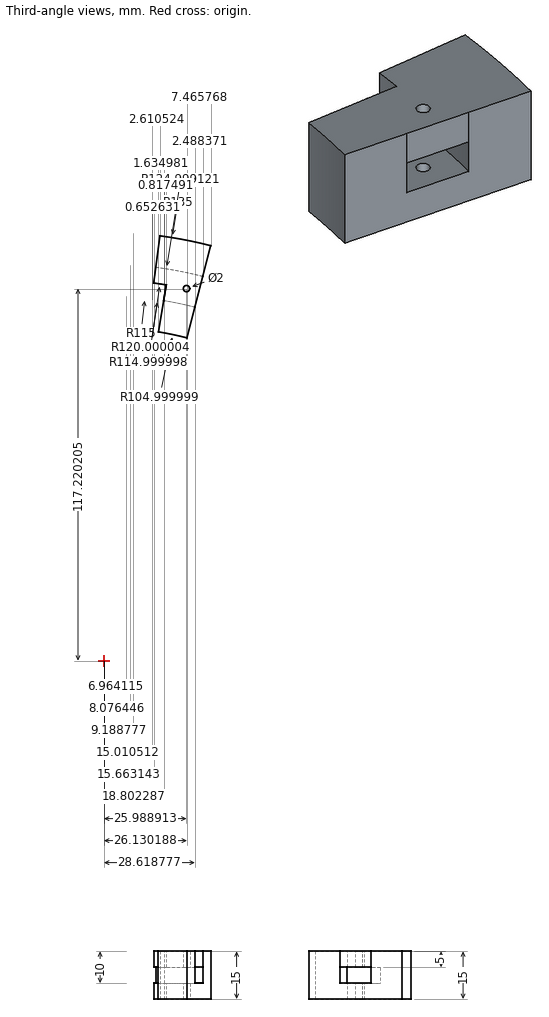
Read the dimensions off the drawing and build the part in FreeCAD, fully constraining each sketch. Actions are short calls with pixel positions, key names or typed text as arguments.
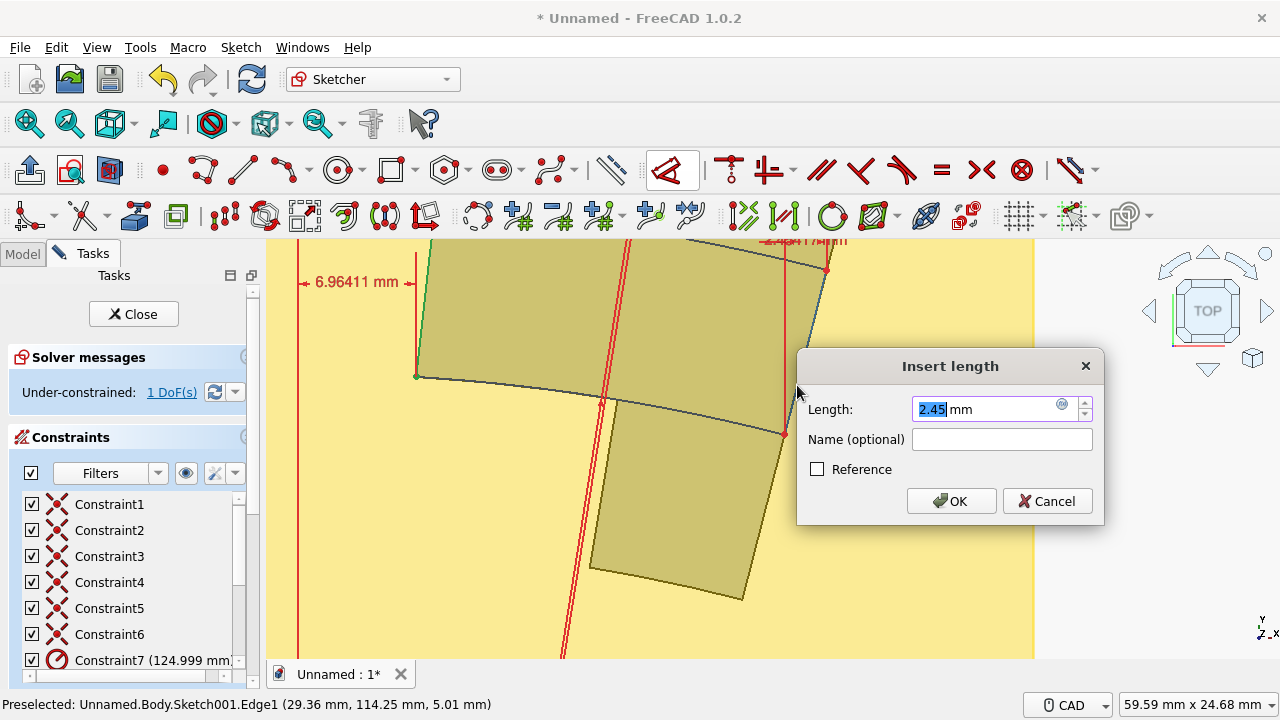
text(2.488371)
key(Return)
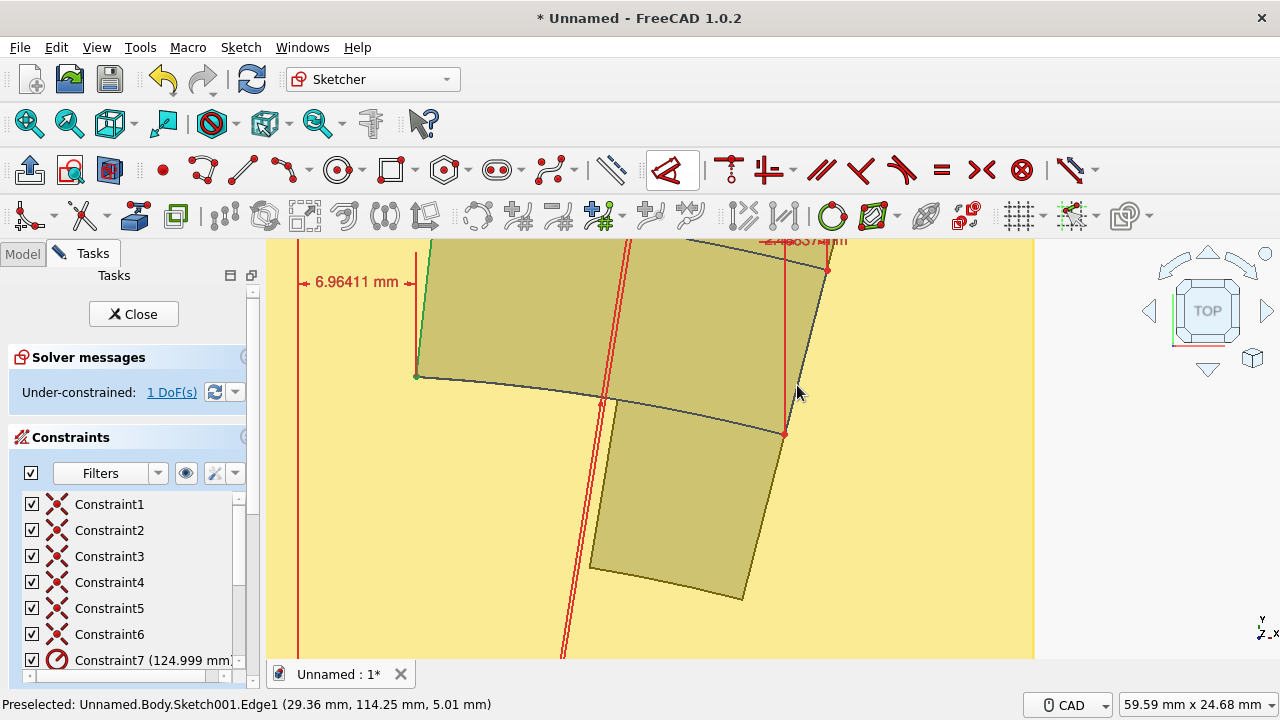
click(785, 435)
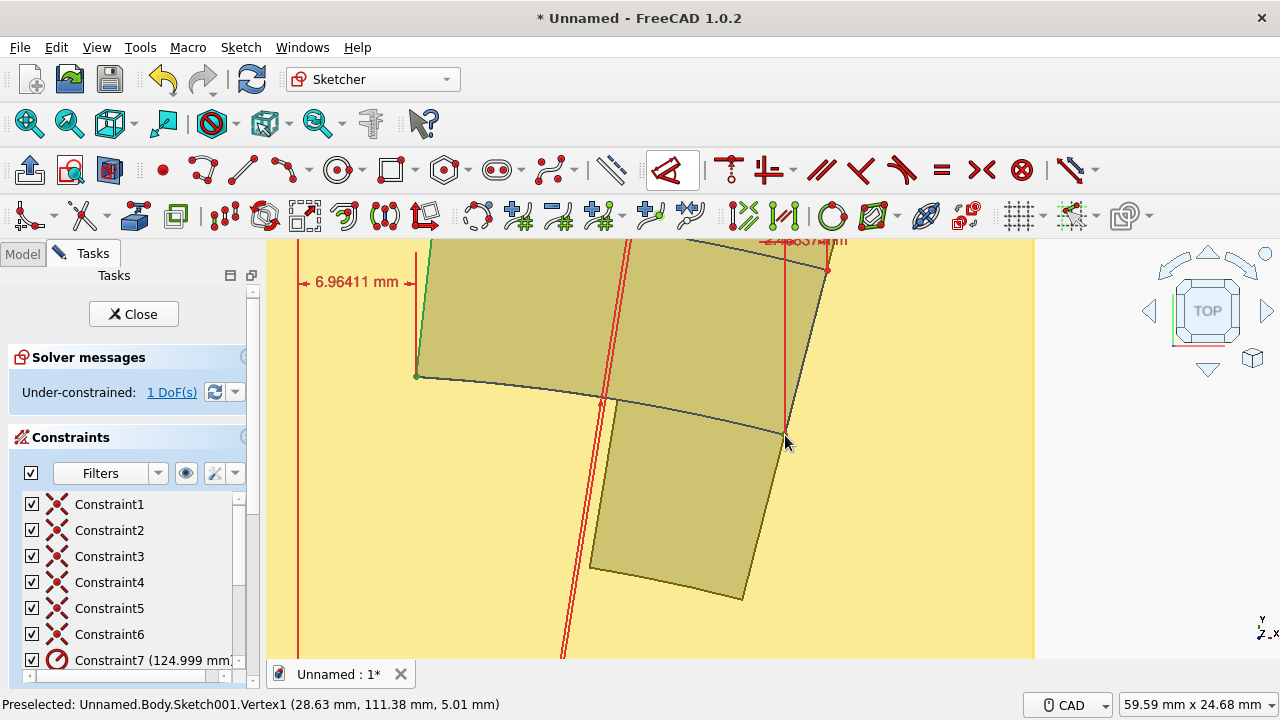
click(694, 170)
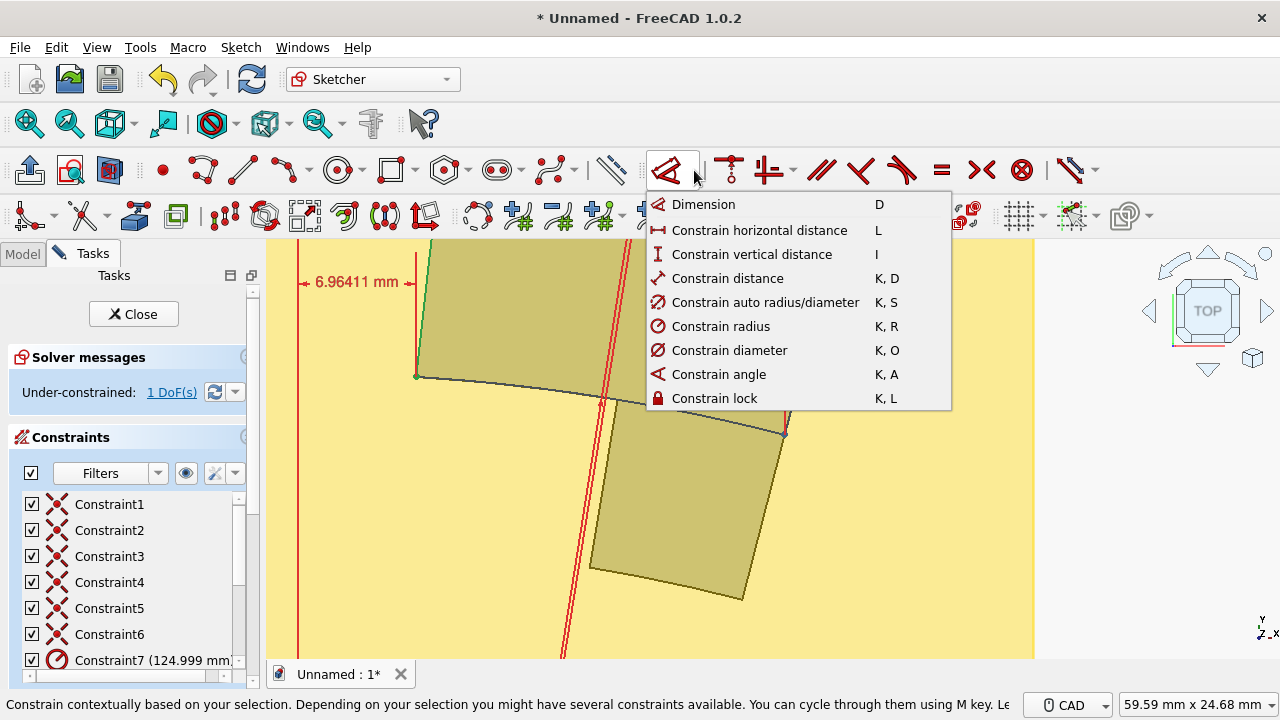
click(799, 230)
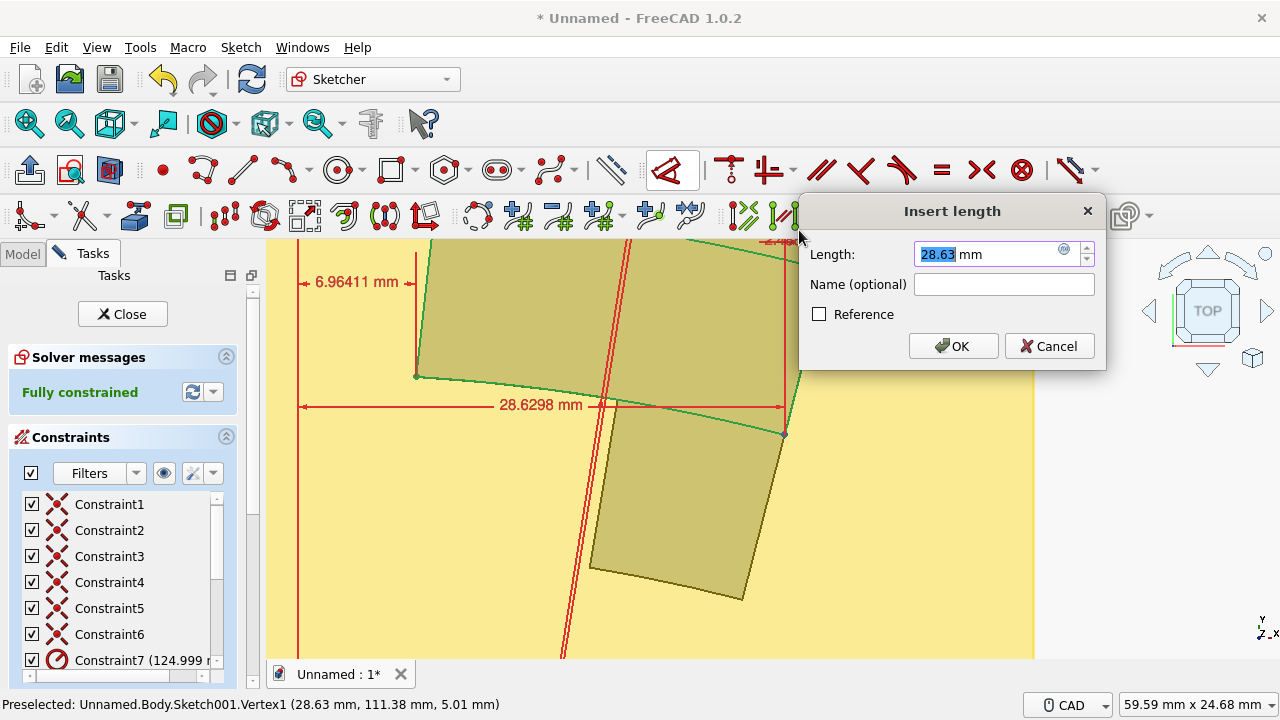
text(28.618777)
key(Return)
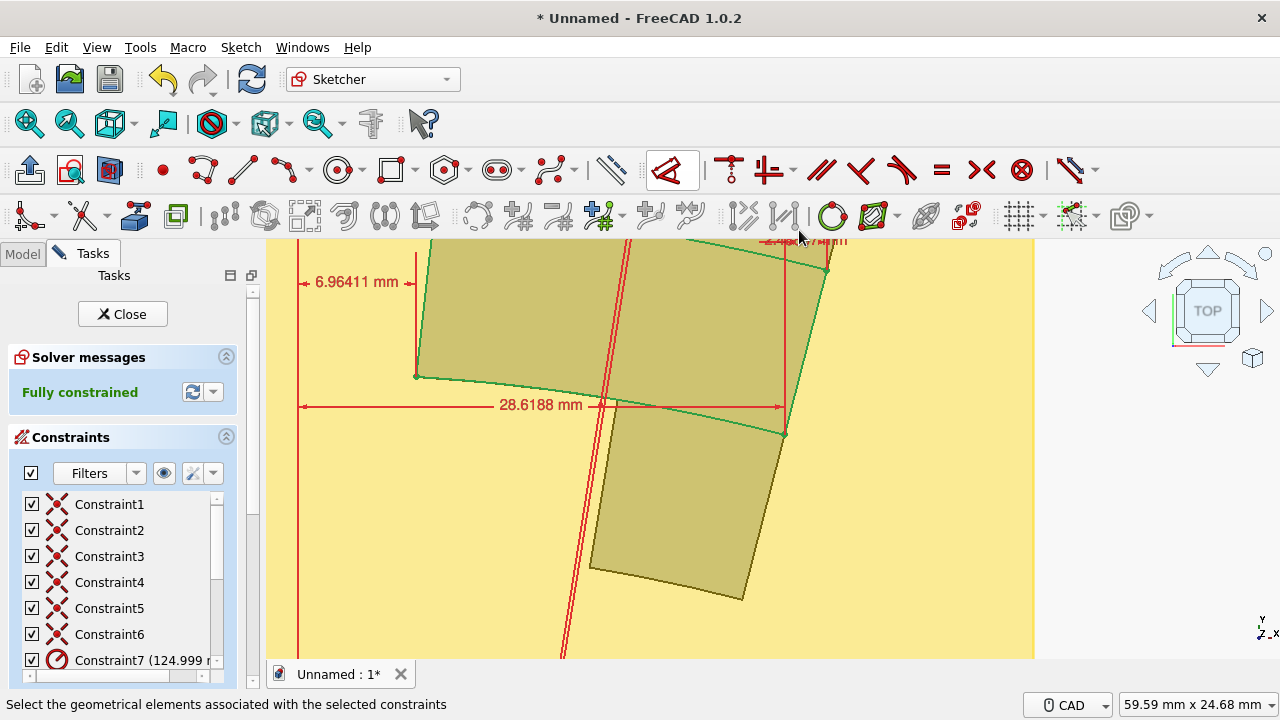
click(123, 314)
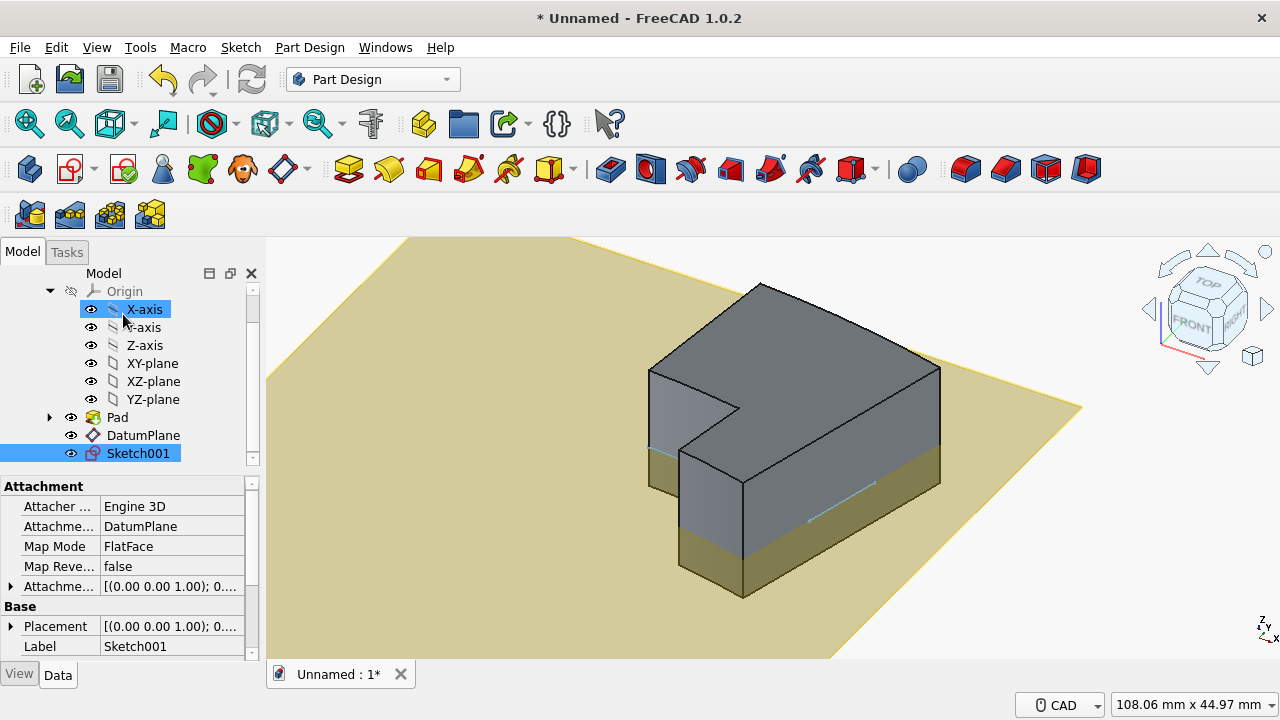
click(612, 170)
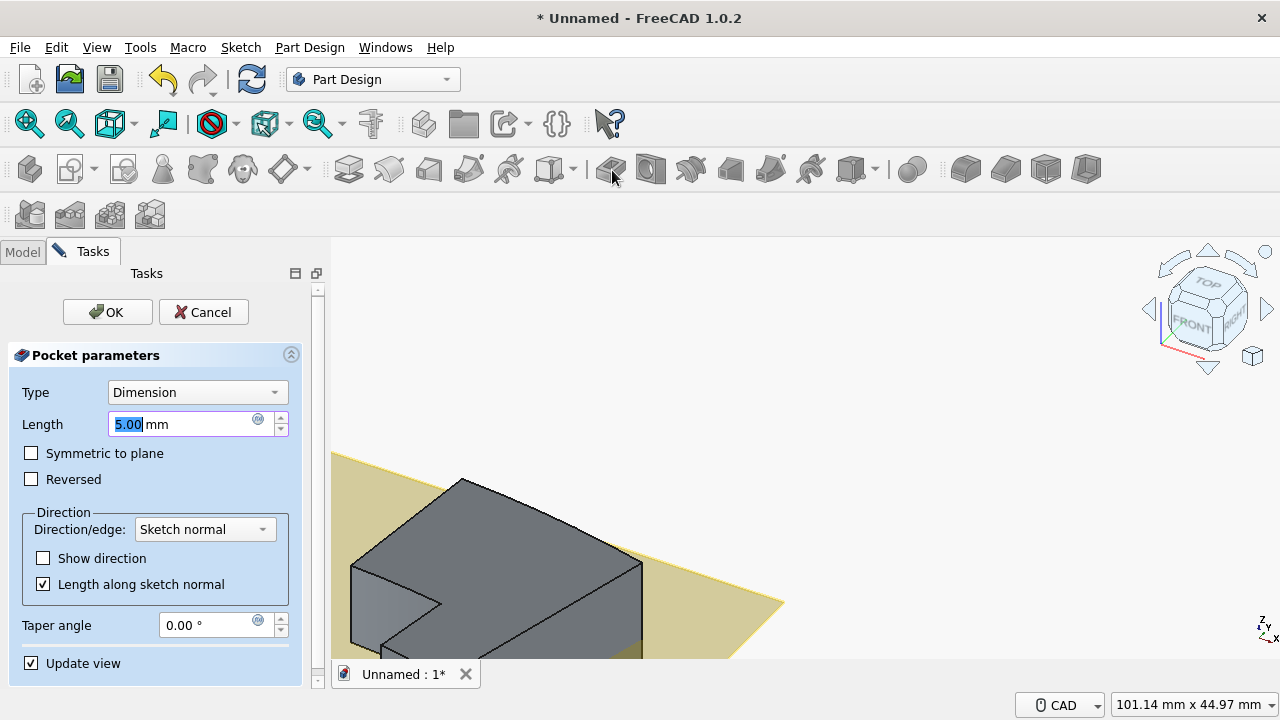
text(10)
key(Tab)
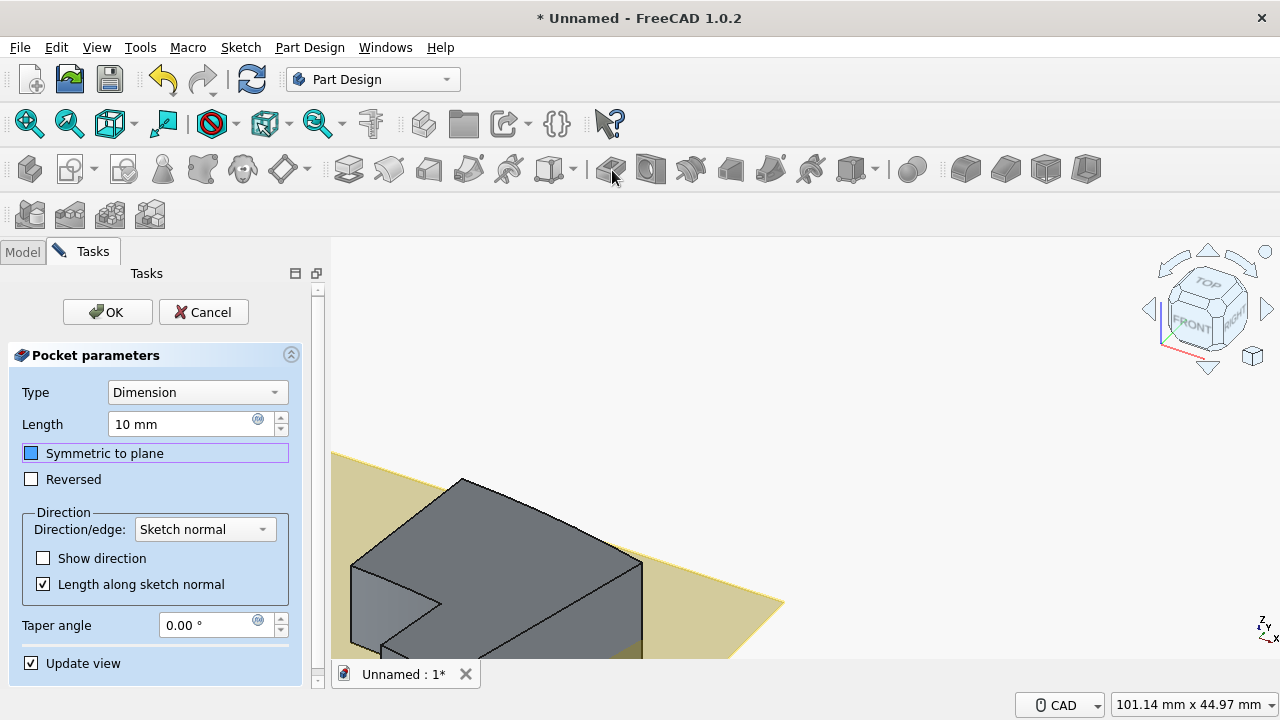
click(30, 479)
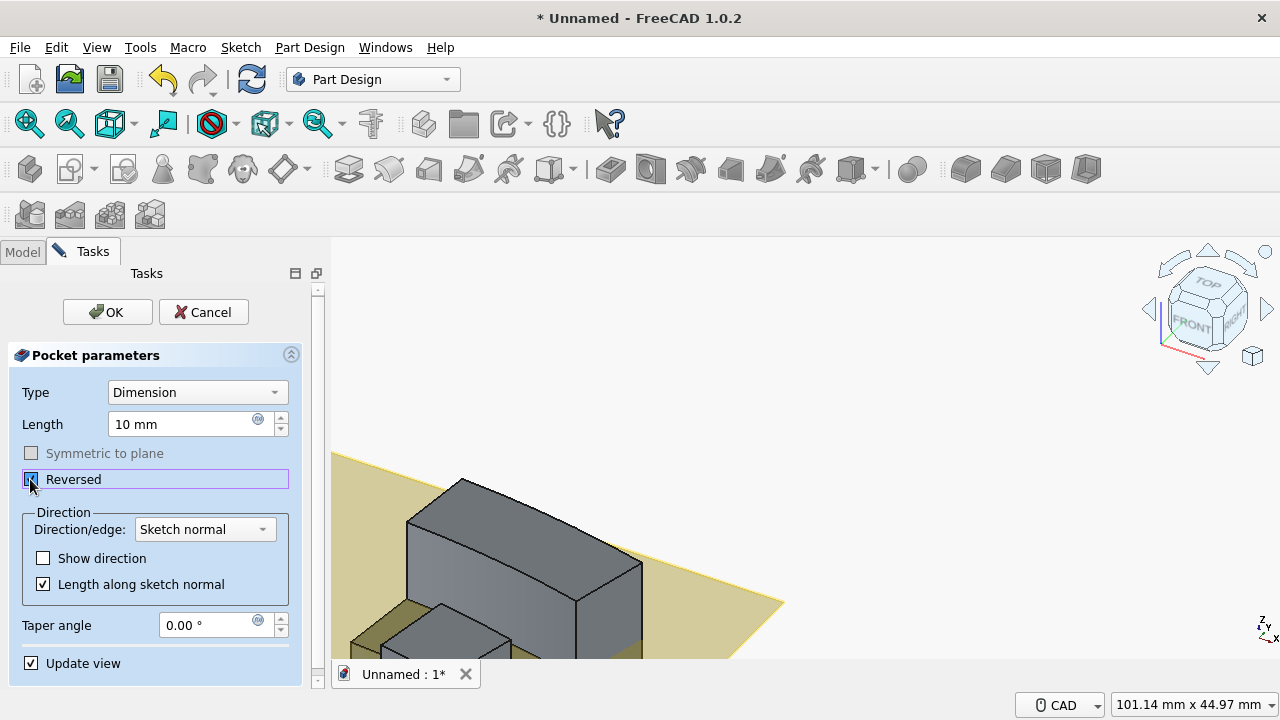
click(108, 312)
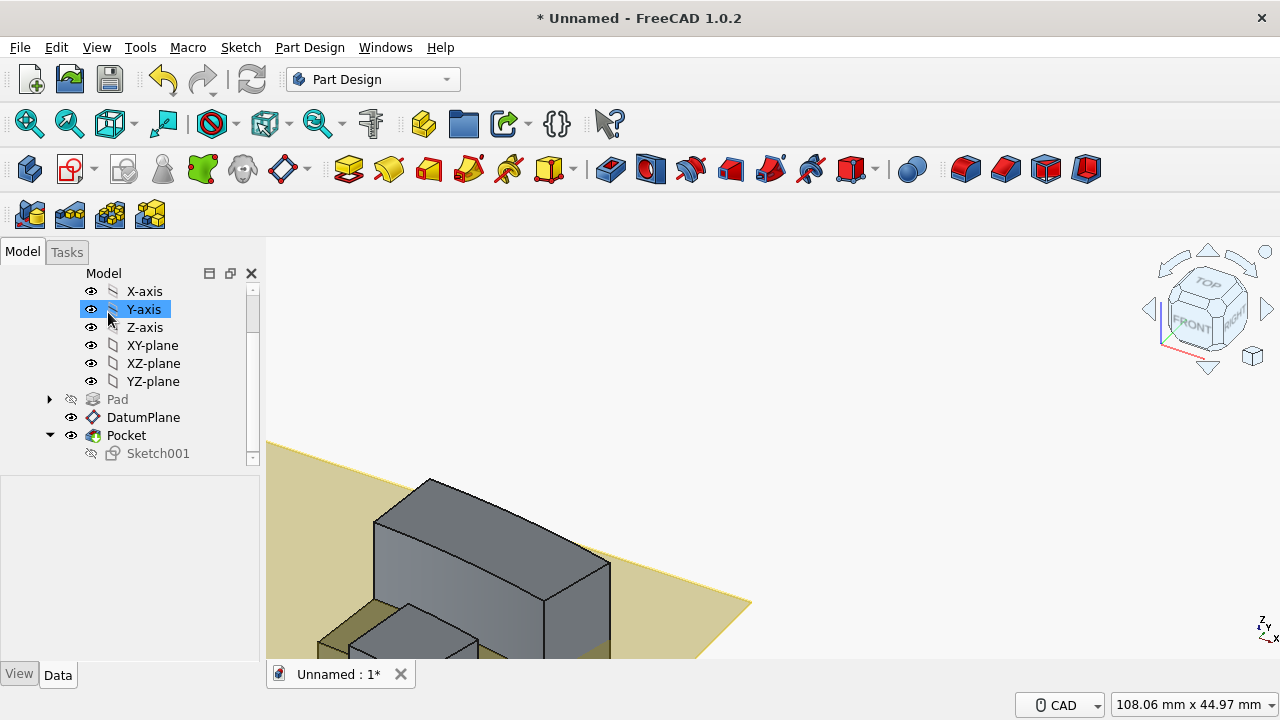
click(116, 417)
key(space)